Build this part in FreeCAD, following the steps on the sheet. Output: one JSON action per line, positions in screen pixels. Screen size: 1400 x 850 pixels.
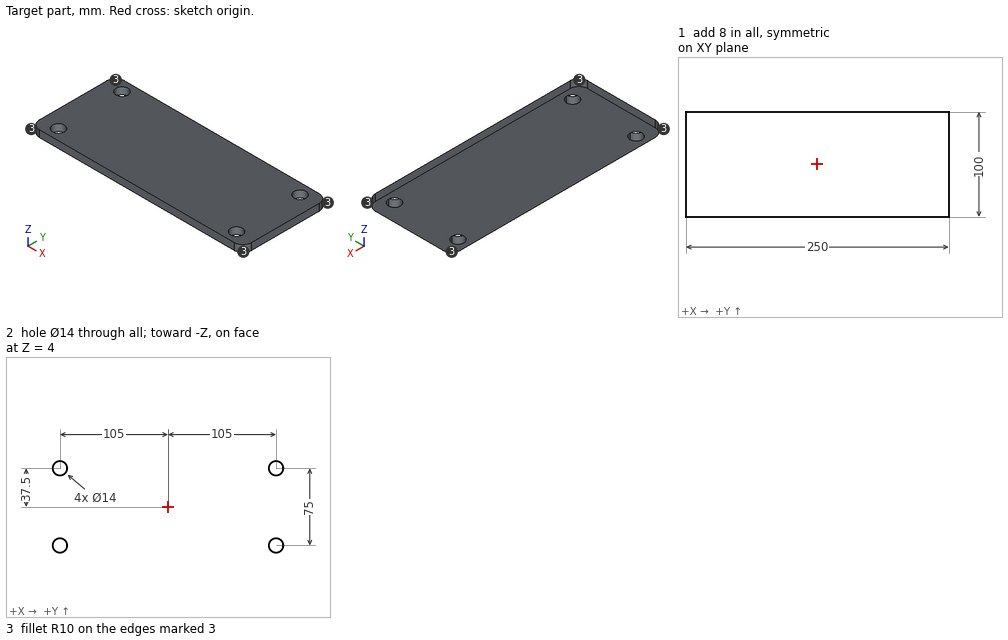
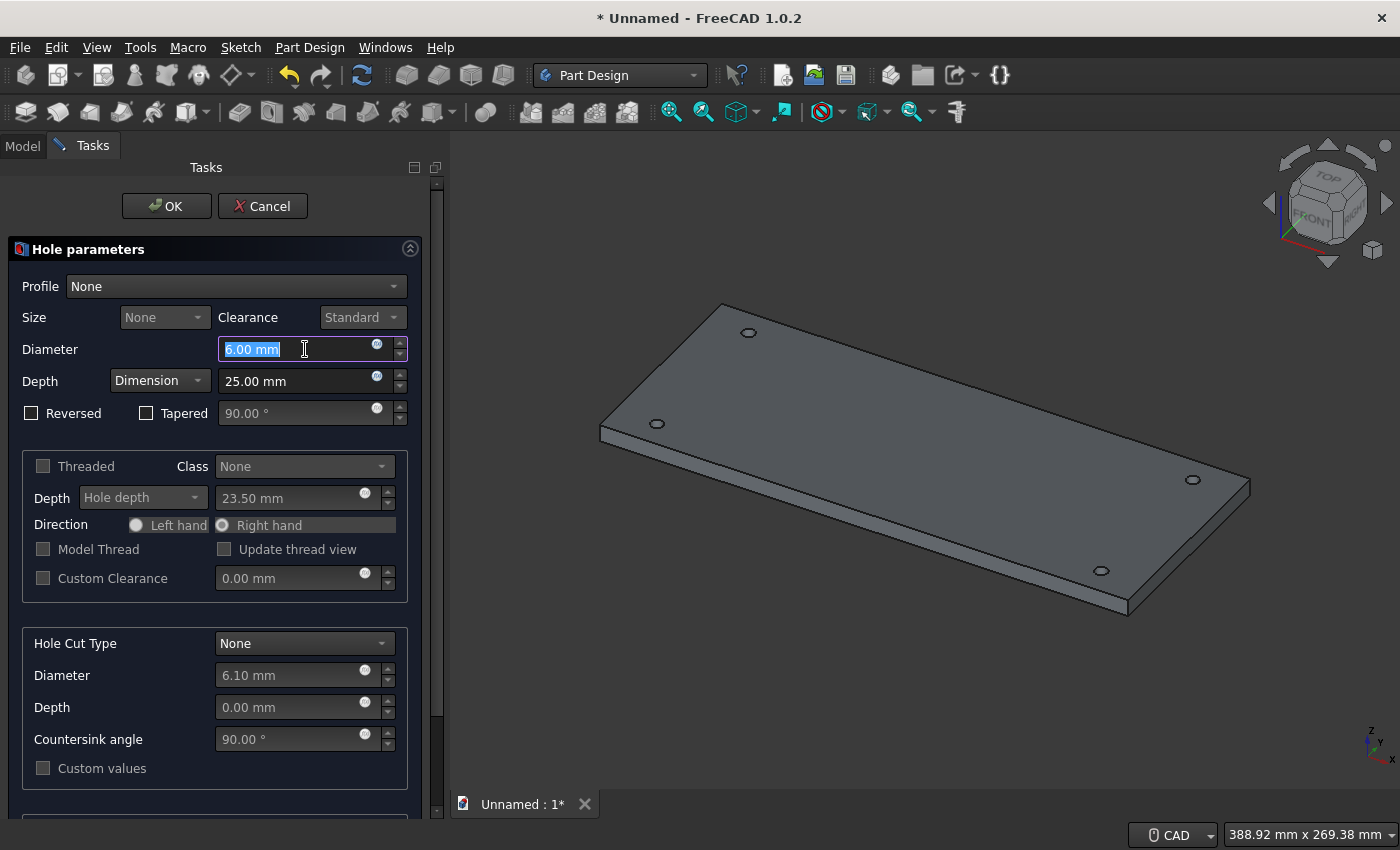
{"action": "type", "text": "14"}
{"action": "key", "text": "Tab"}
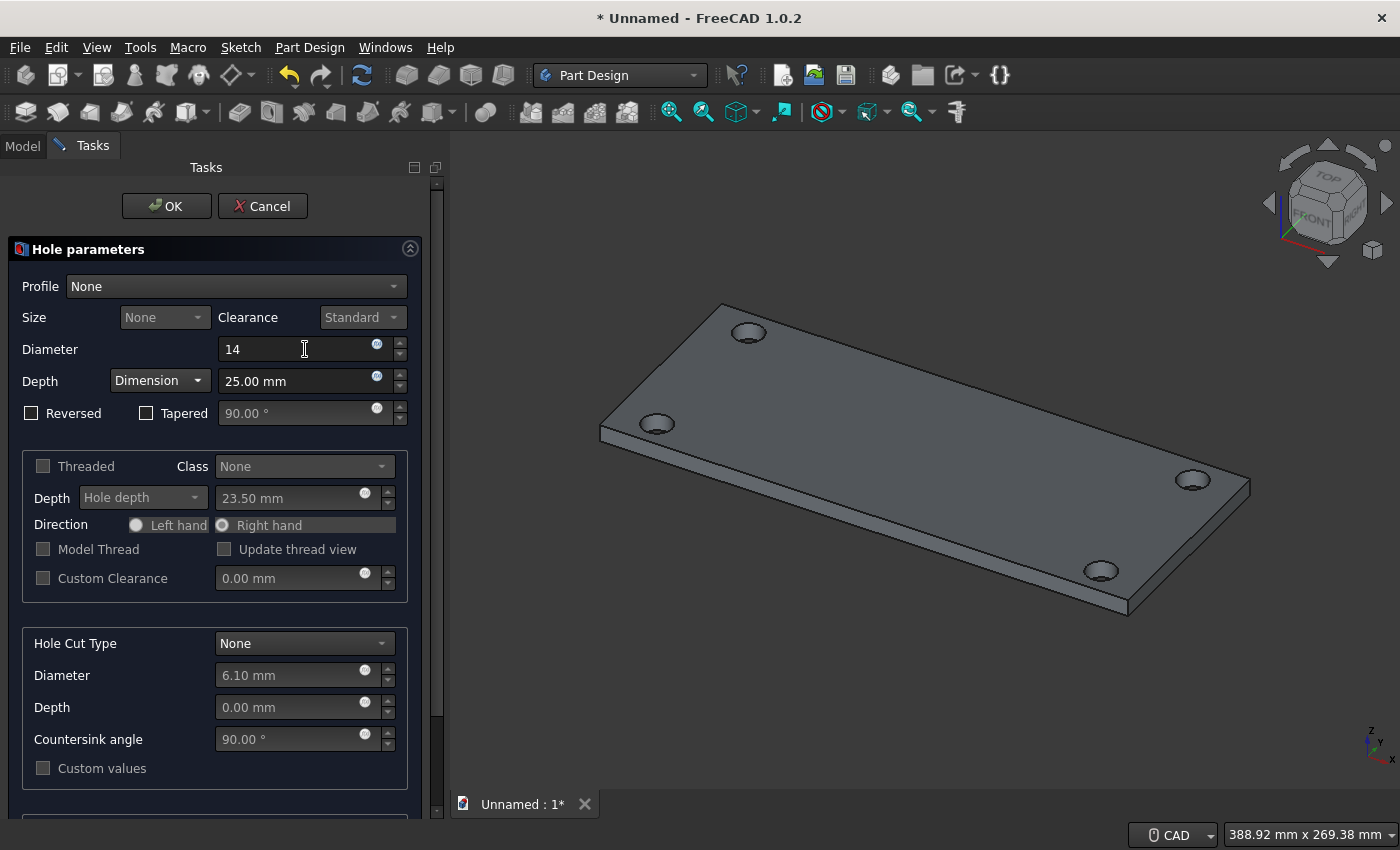
{"action": "left_click", "coordinate": [161, 380]}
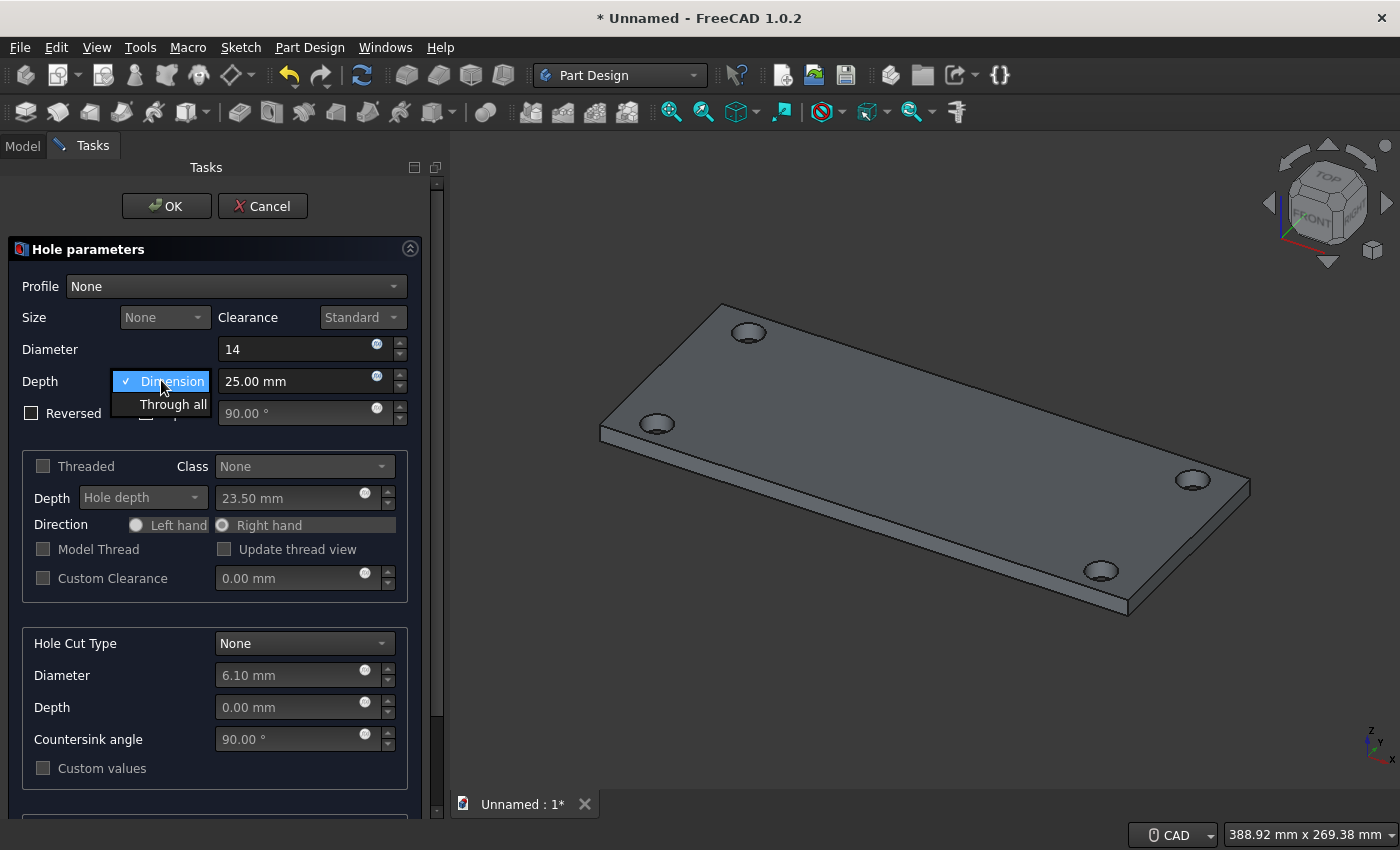
{"action": "left_click", "coordinate": [160, 404]}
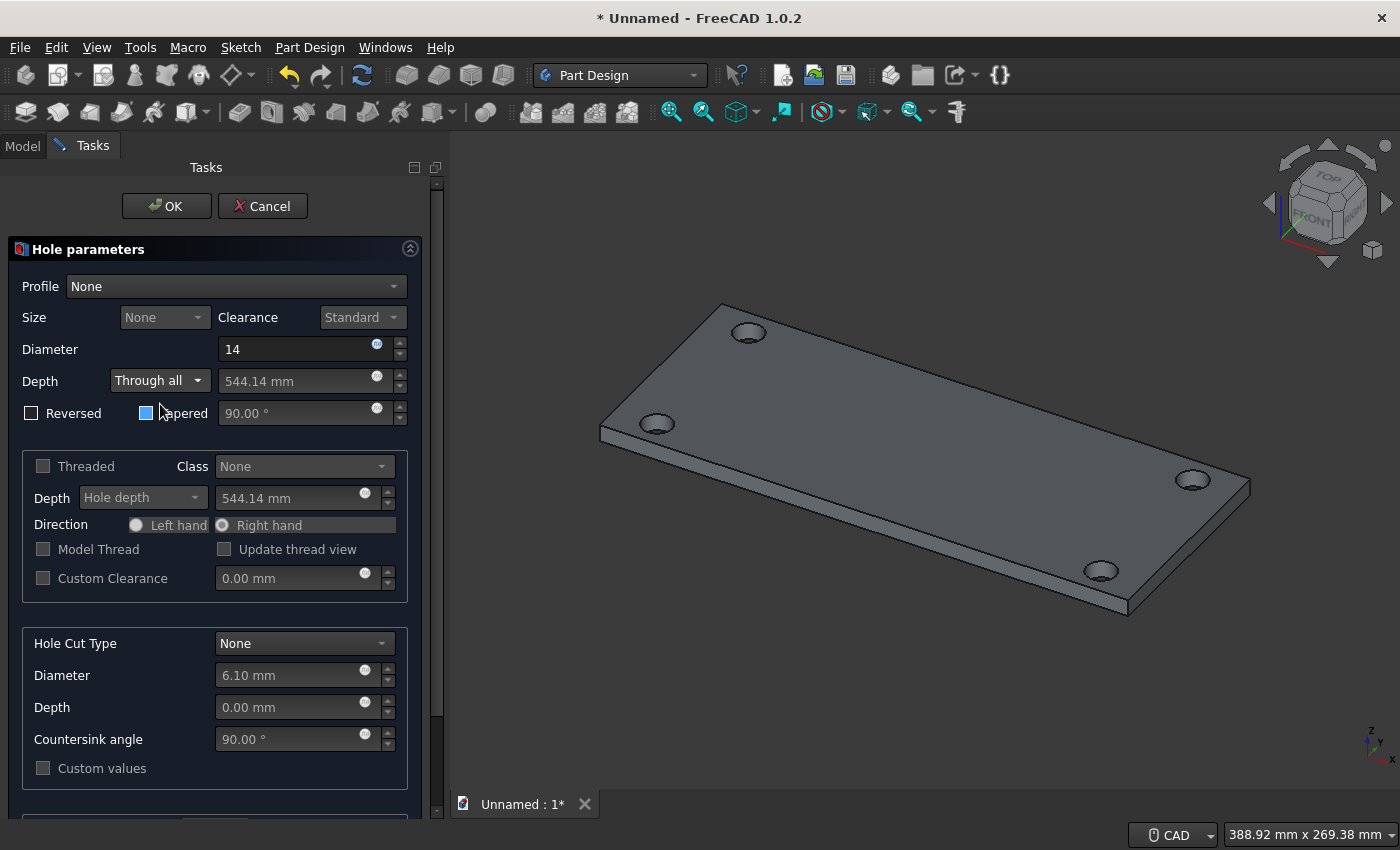
{"action": "left_click", "coordinate": [167, 206]}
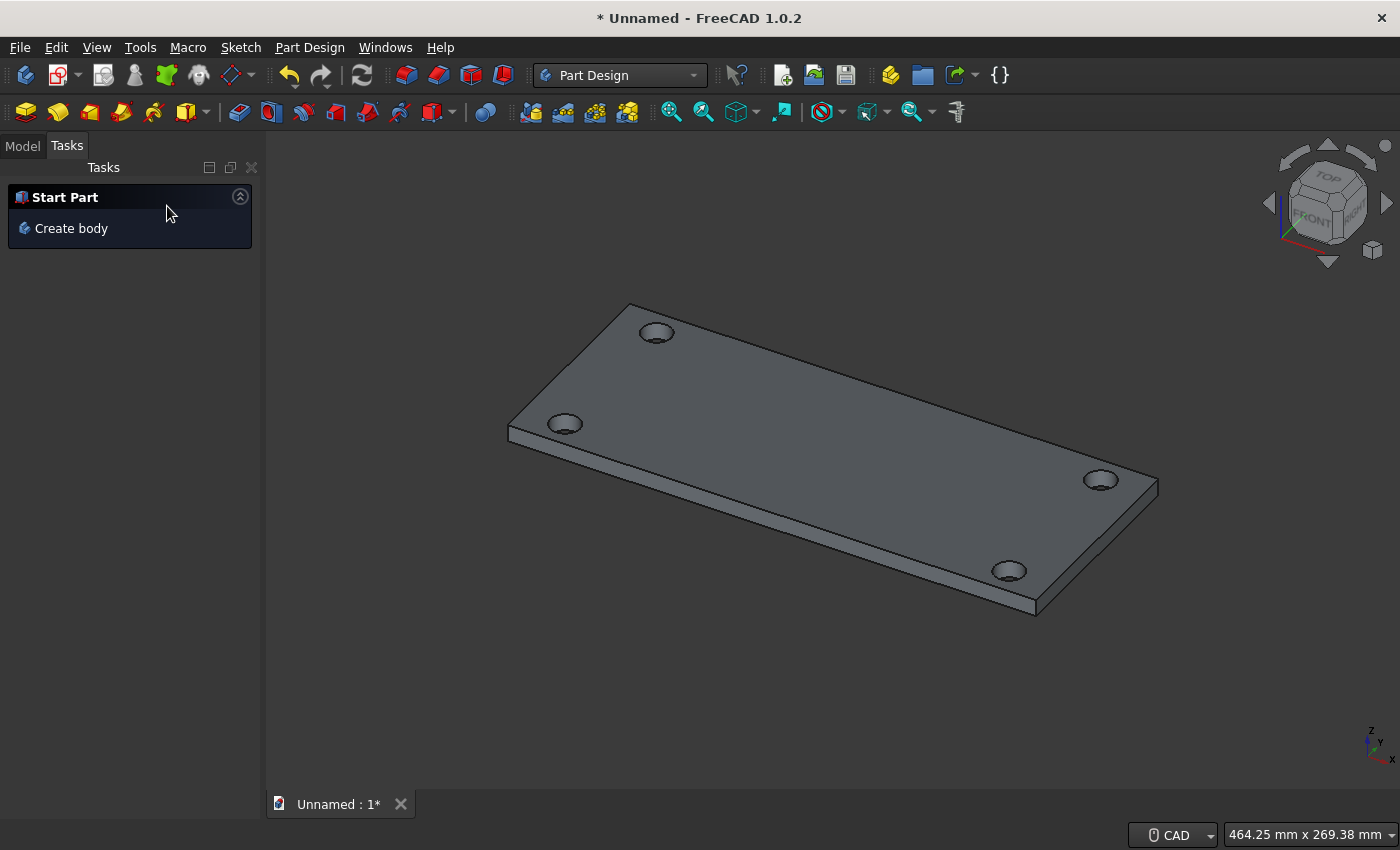
{"action": "left_click", "coordinate": [1036, 607]}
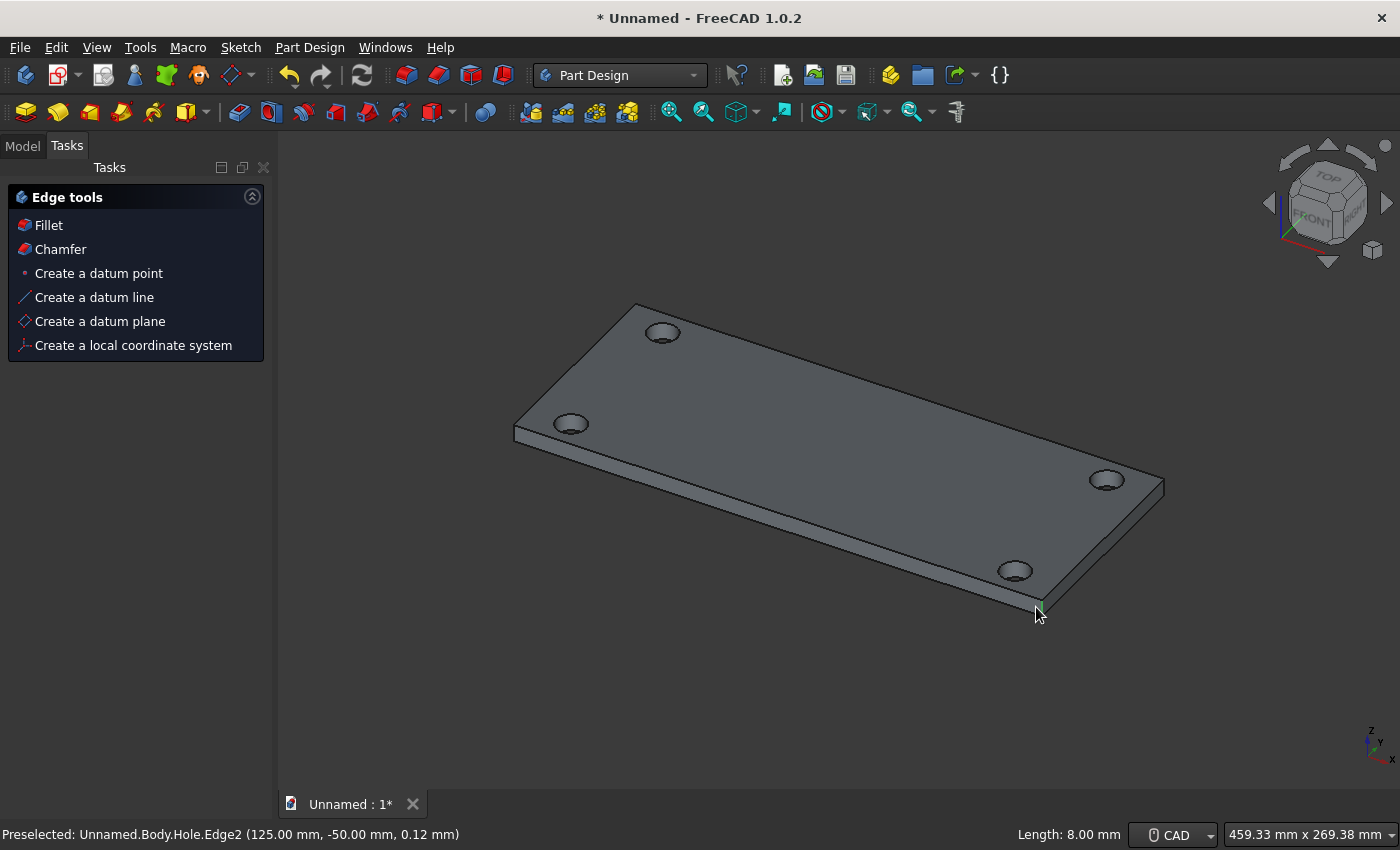
{"action": "scroll", "coordinate": [636, 311], "scroll_direction": "up", "scroll_amount": 4}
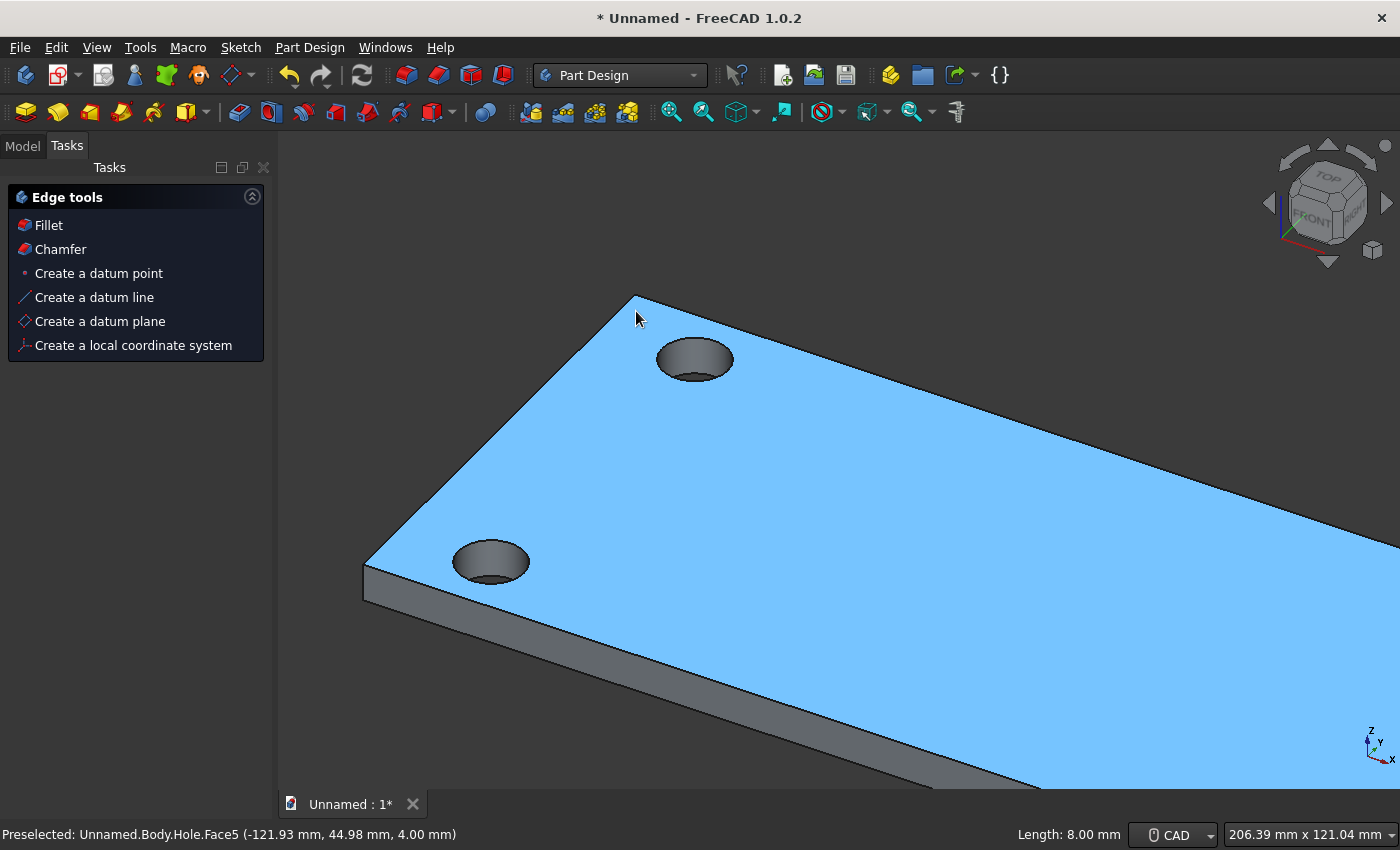
{"action": "left_click", "coordinate": [672, 112]}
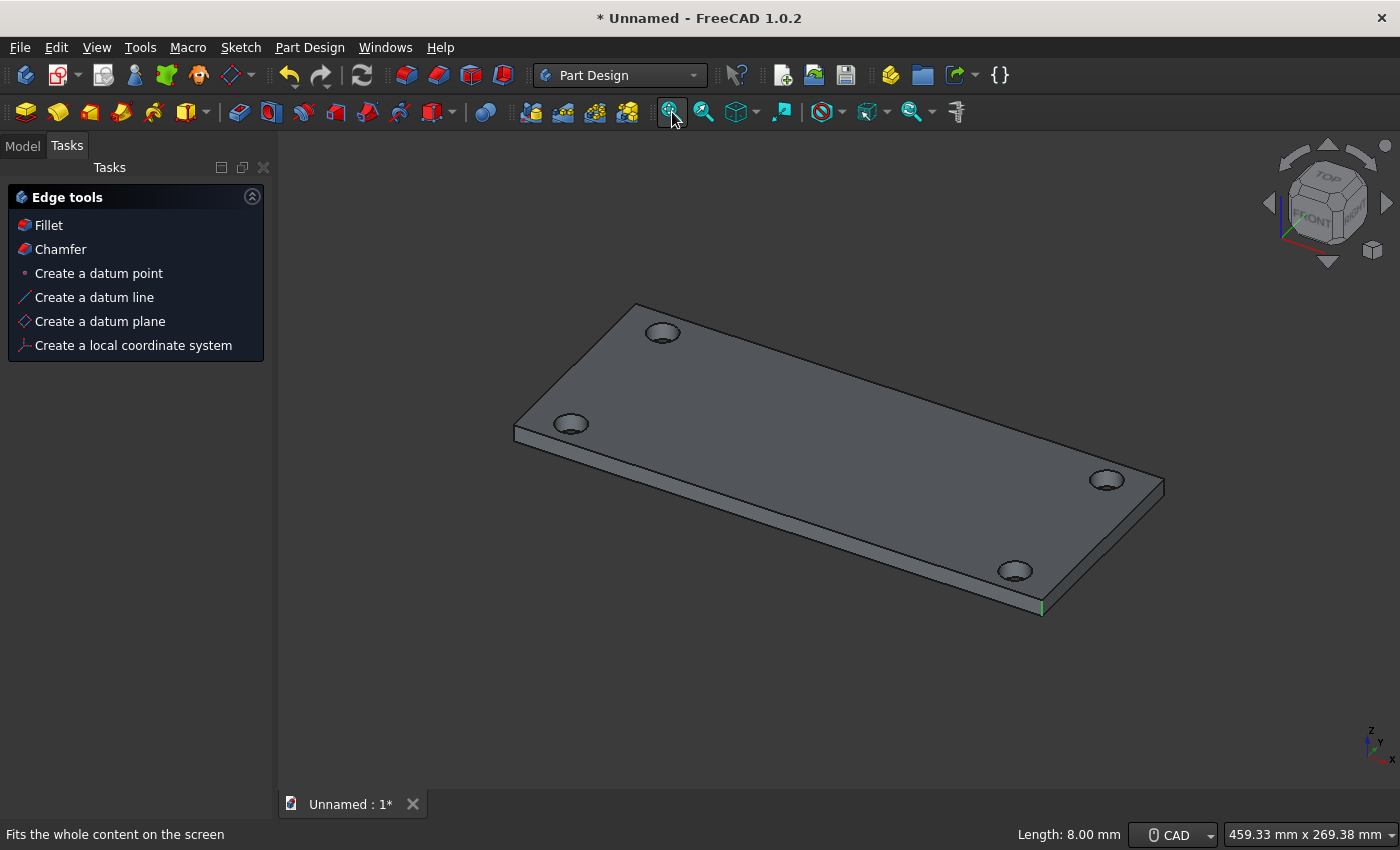
{"action": "key", "text": "0"}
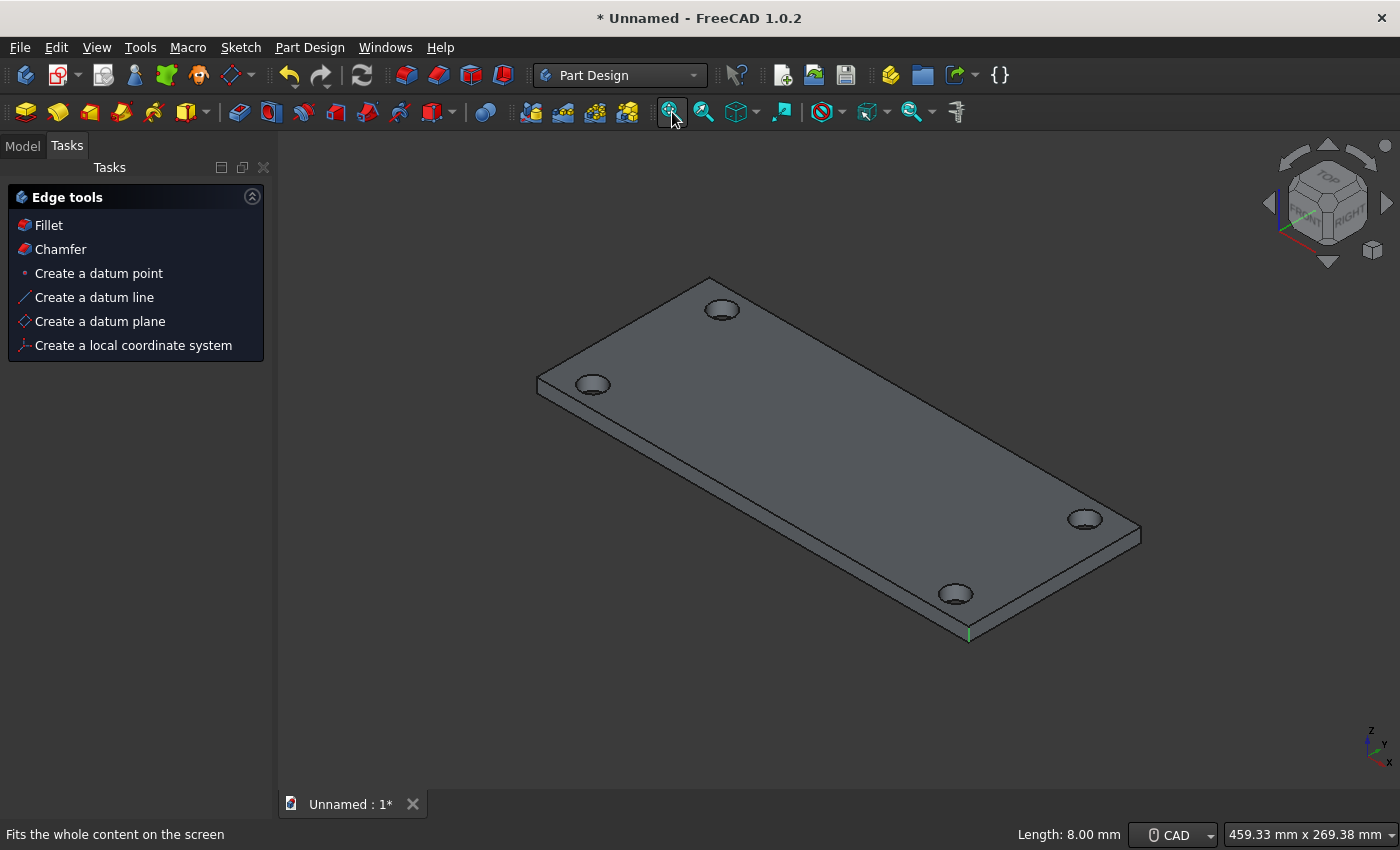
{"action": "scroll", "coordinate": [709, 284], "scroll_direction": "up", "scroll_amount": 4}